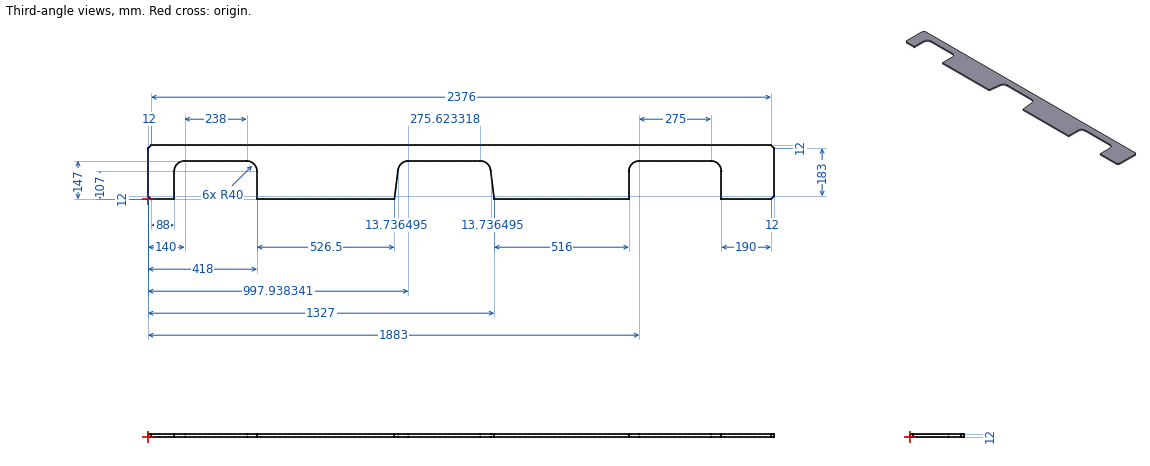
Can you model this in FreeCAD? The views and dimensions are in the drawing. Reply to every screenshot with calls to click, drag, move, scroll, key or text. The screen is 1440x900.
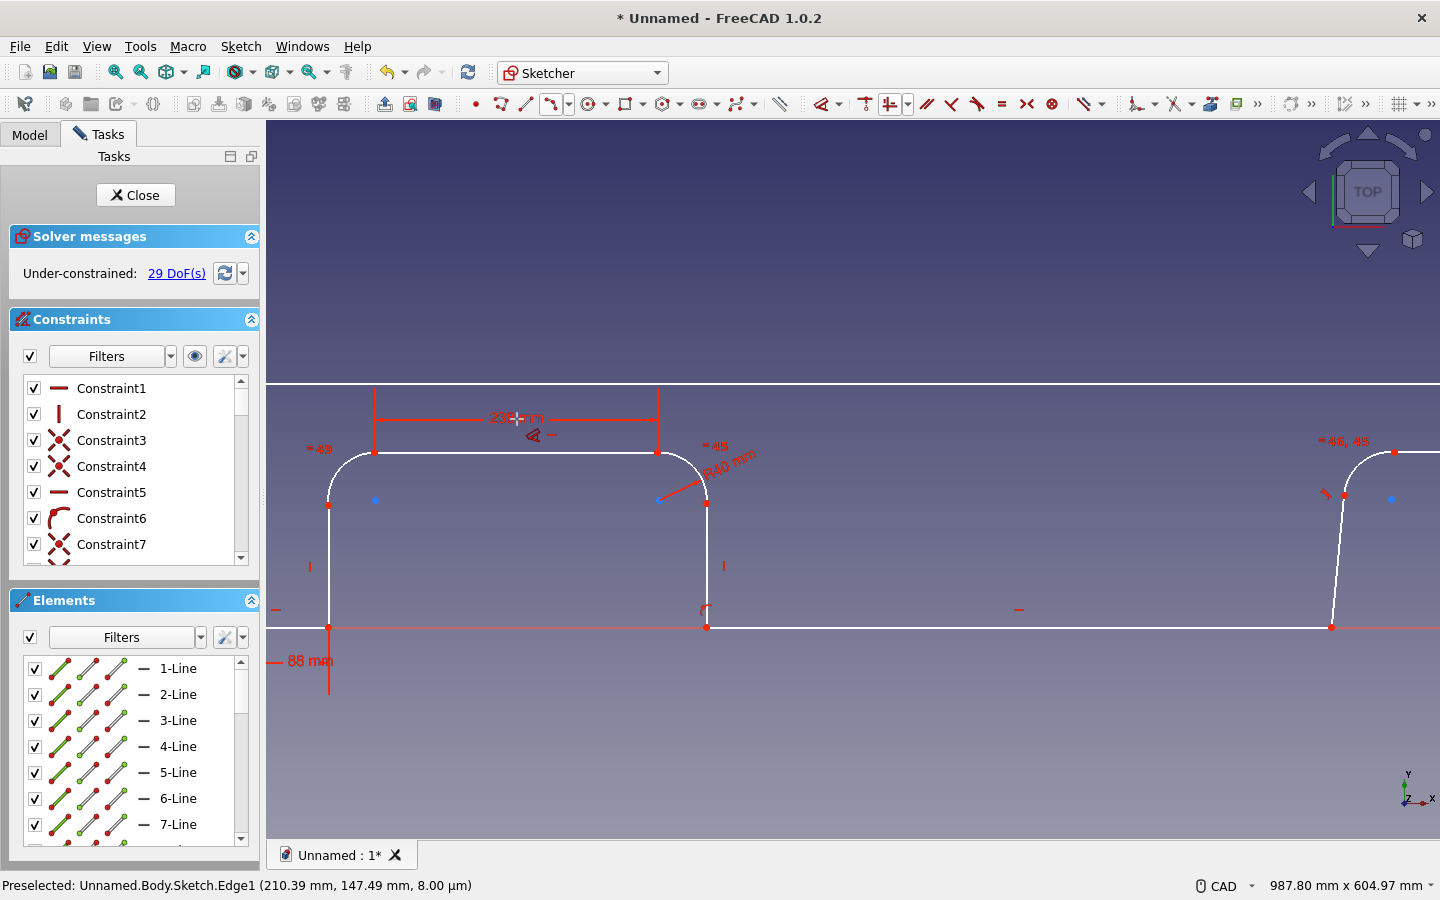
click(707, 540)
click(673, 565)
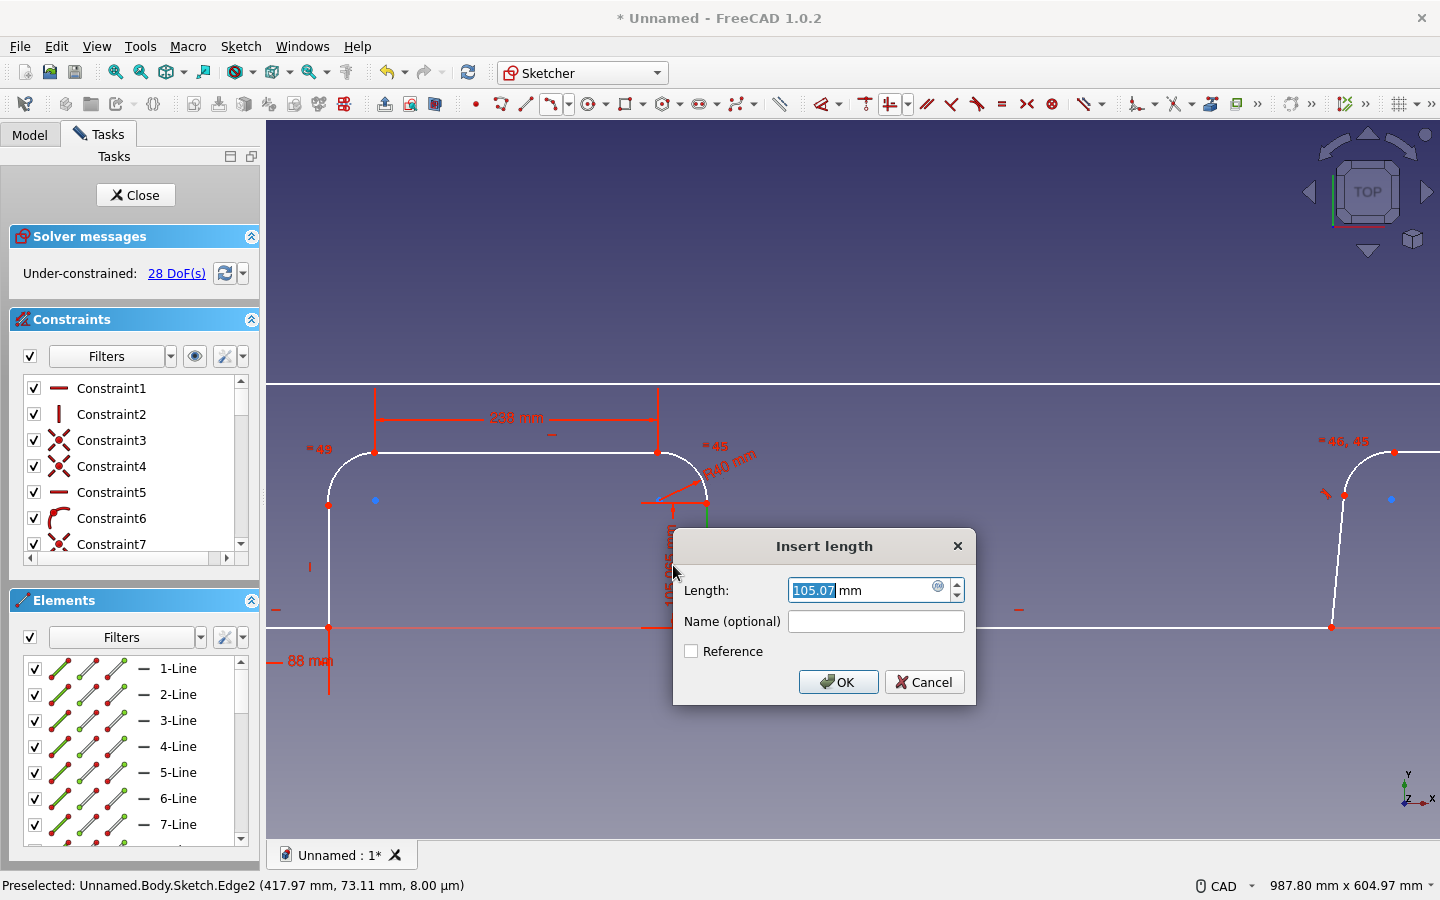
text(107)
key(Return)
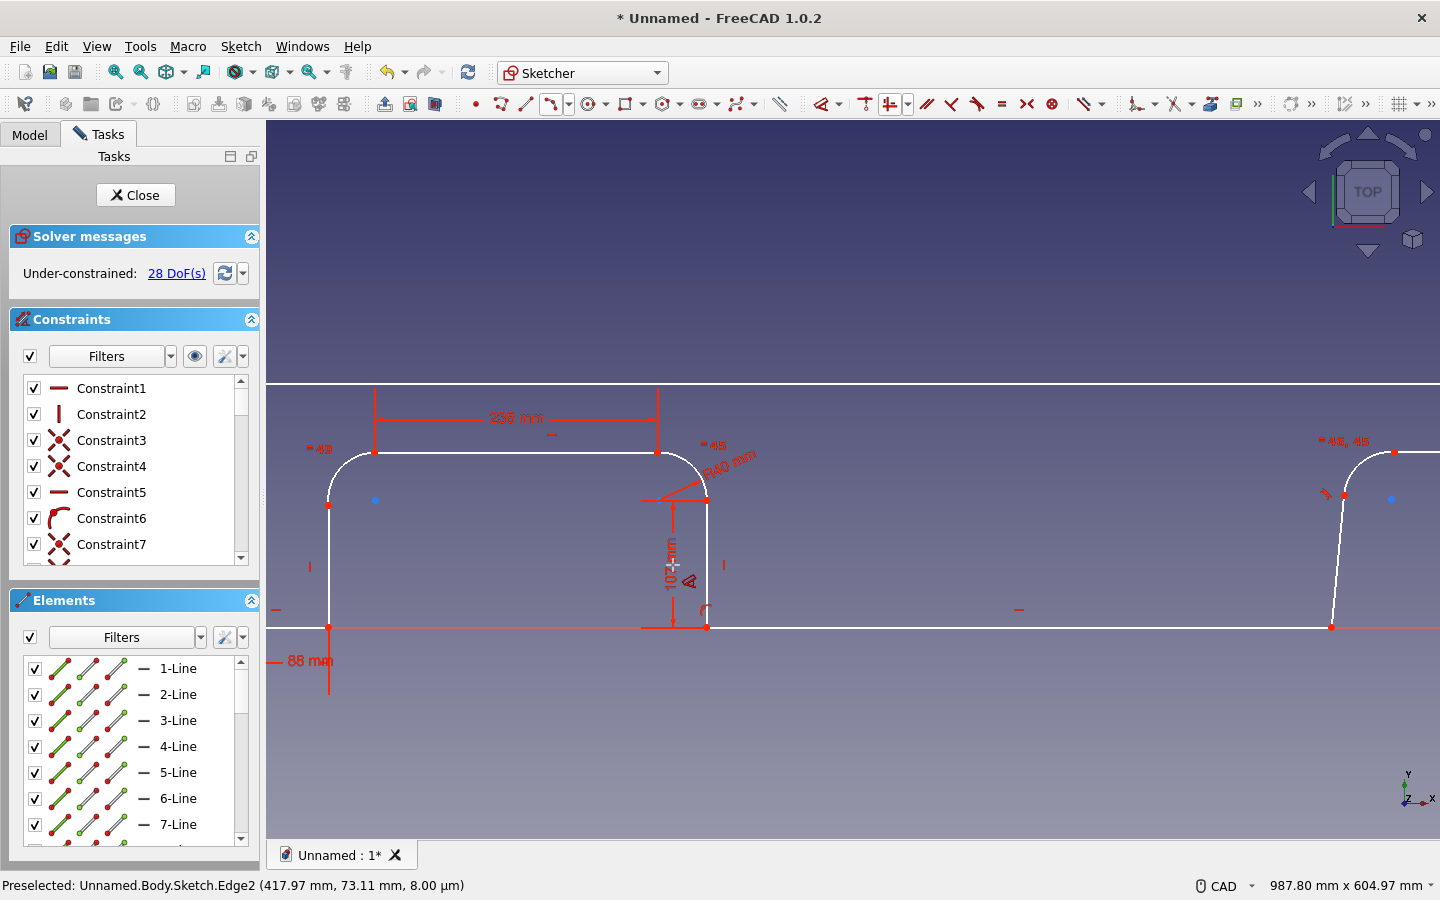
scroll(506, 471, down, 7)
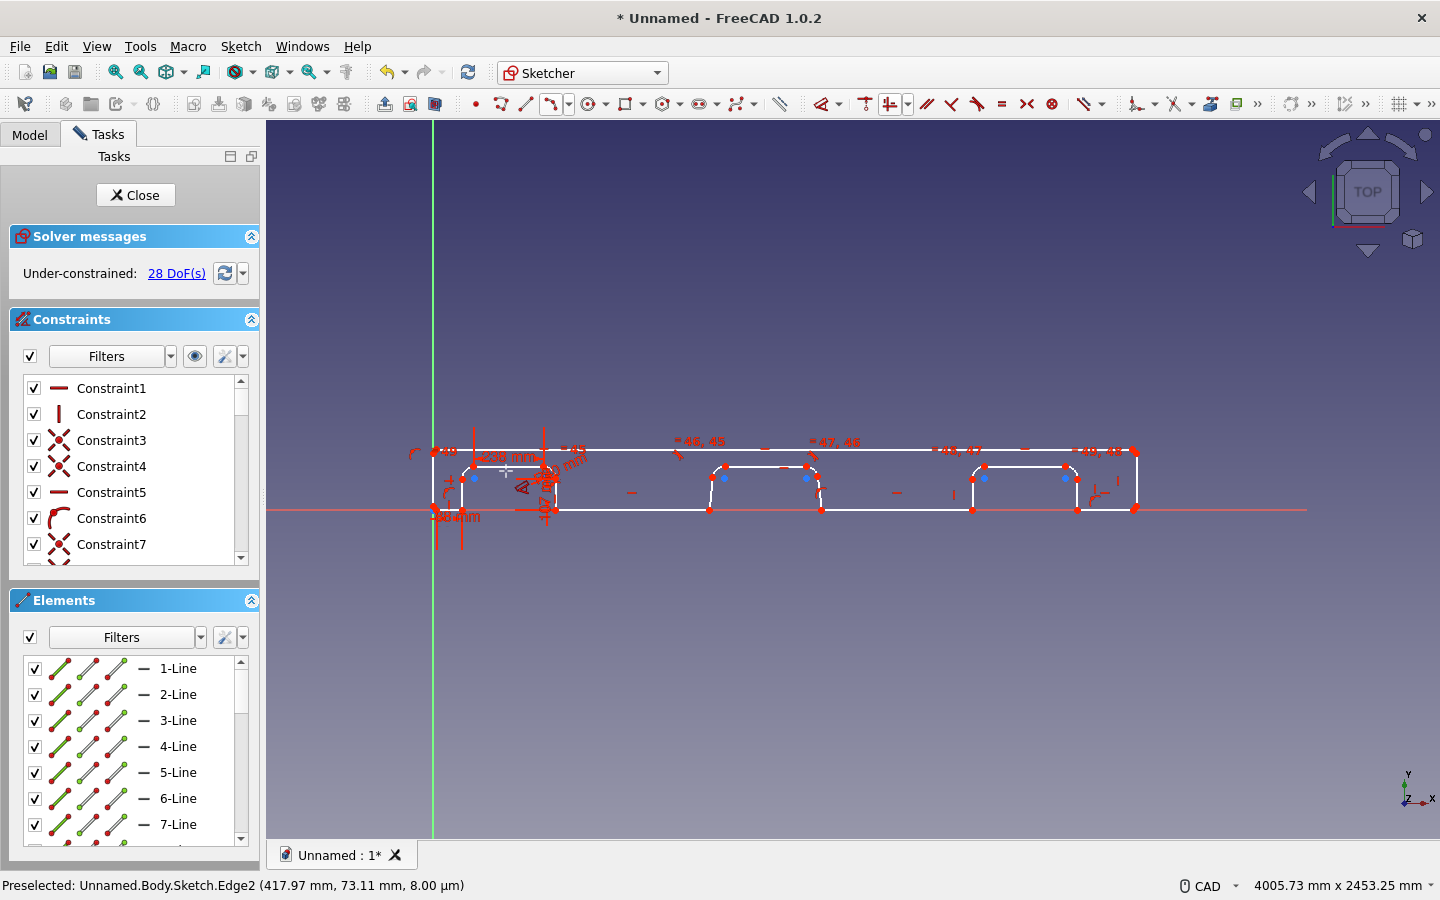
click(867, 510)
click(897, 544)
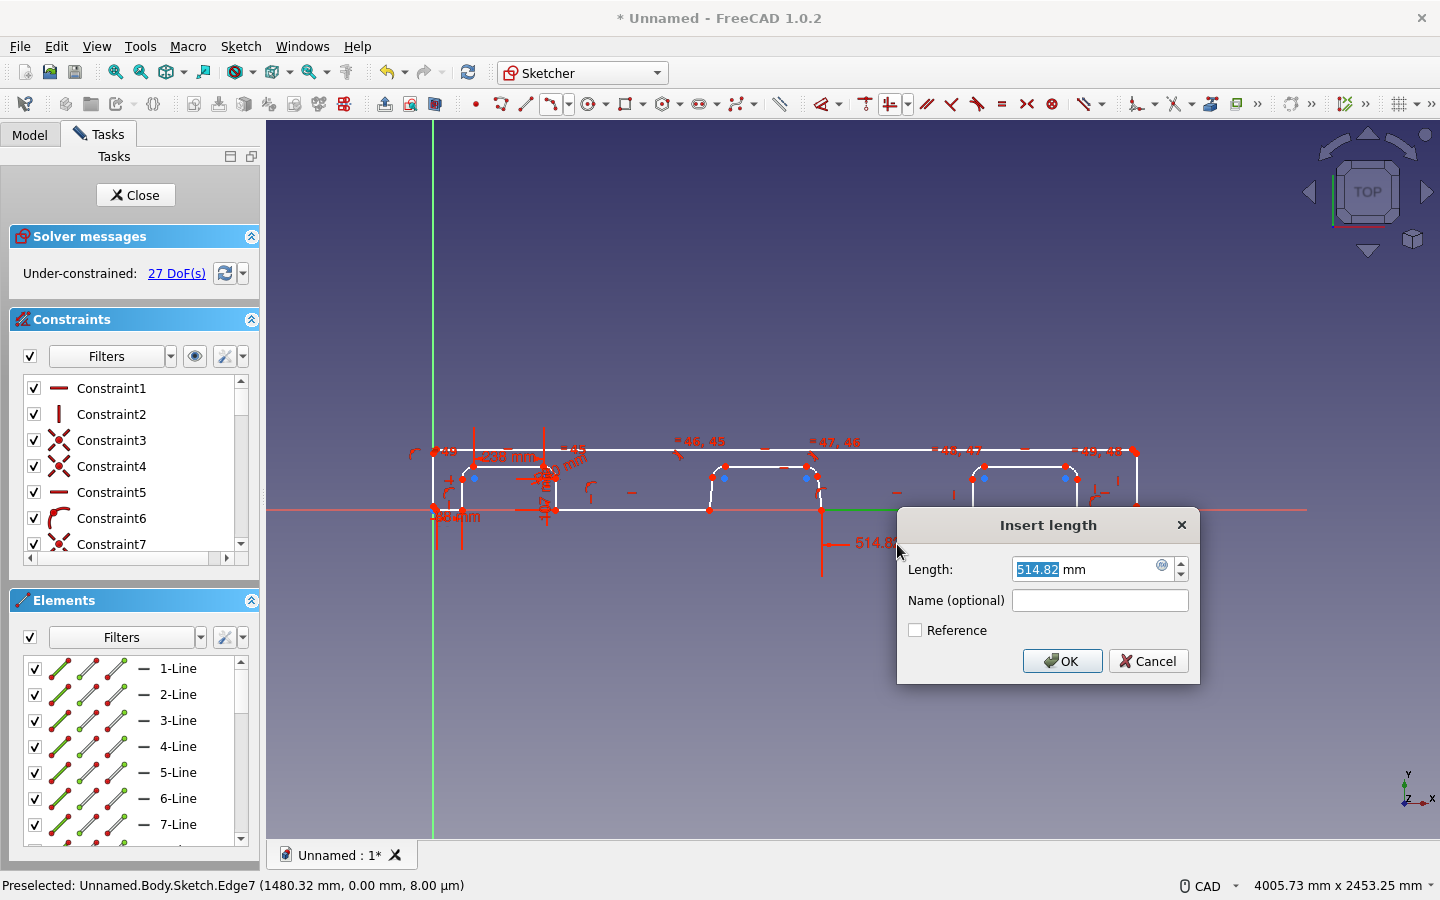
text(516)
key(Return)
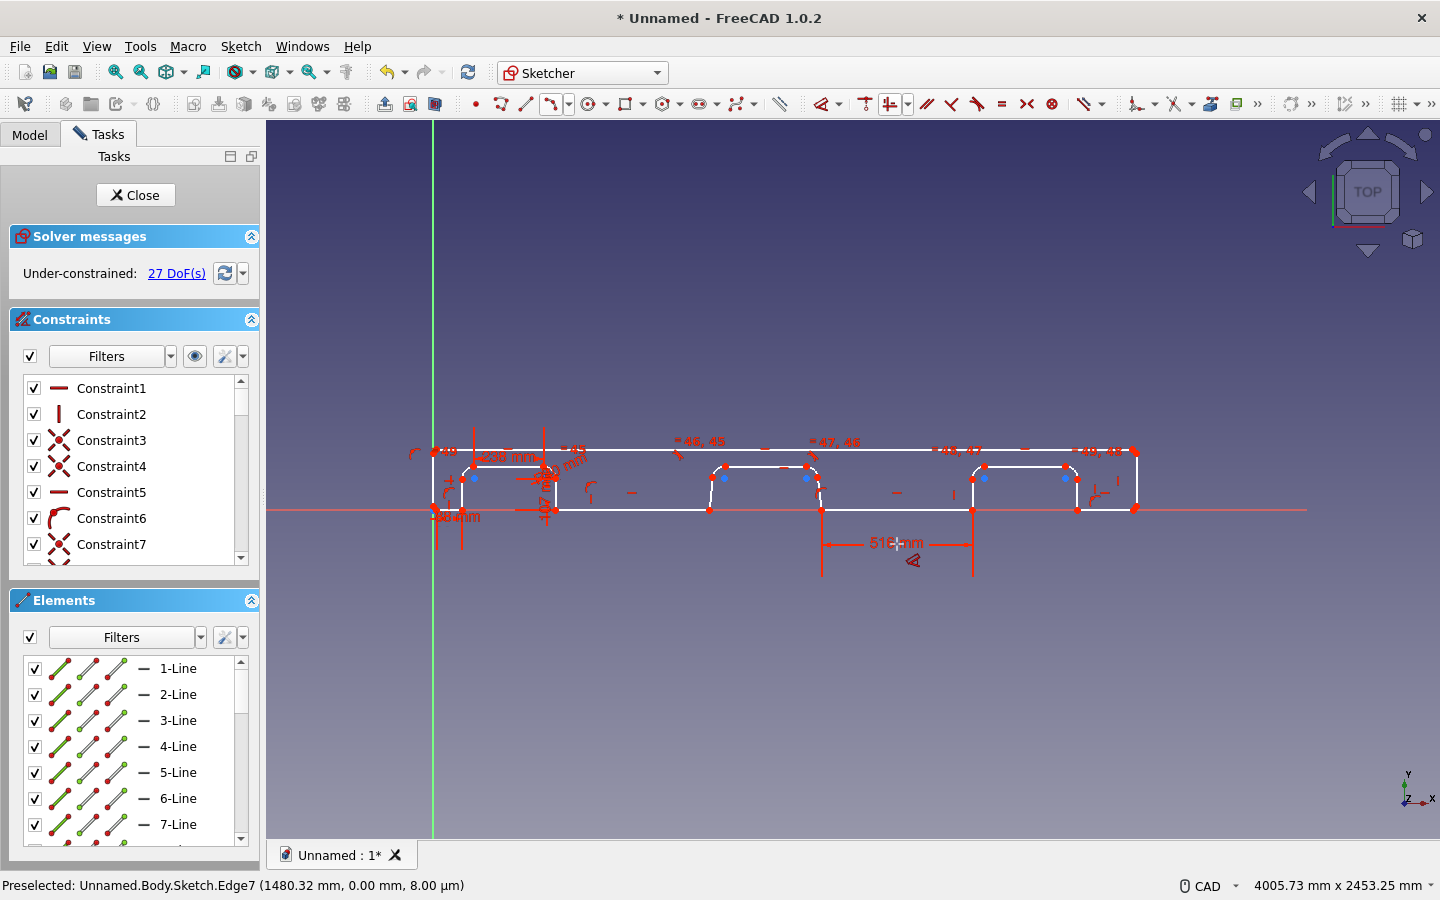
scroll(973, 501, up, 3)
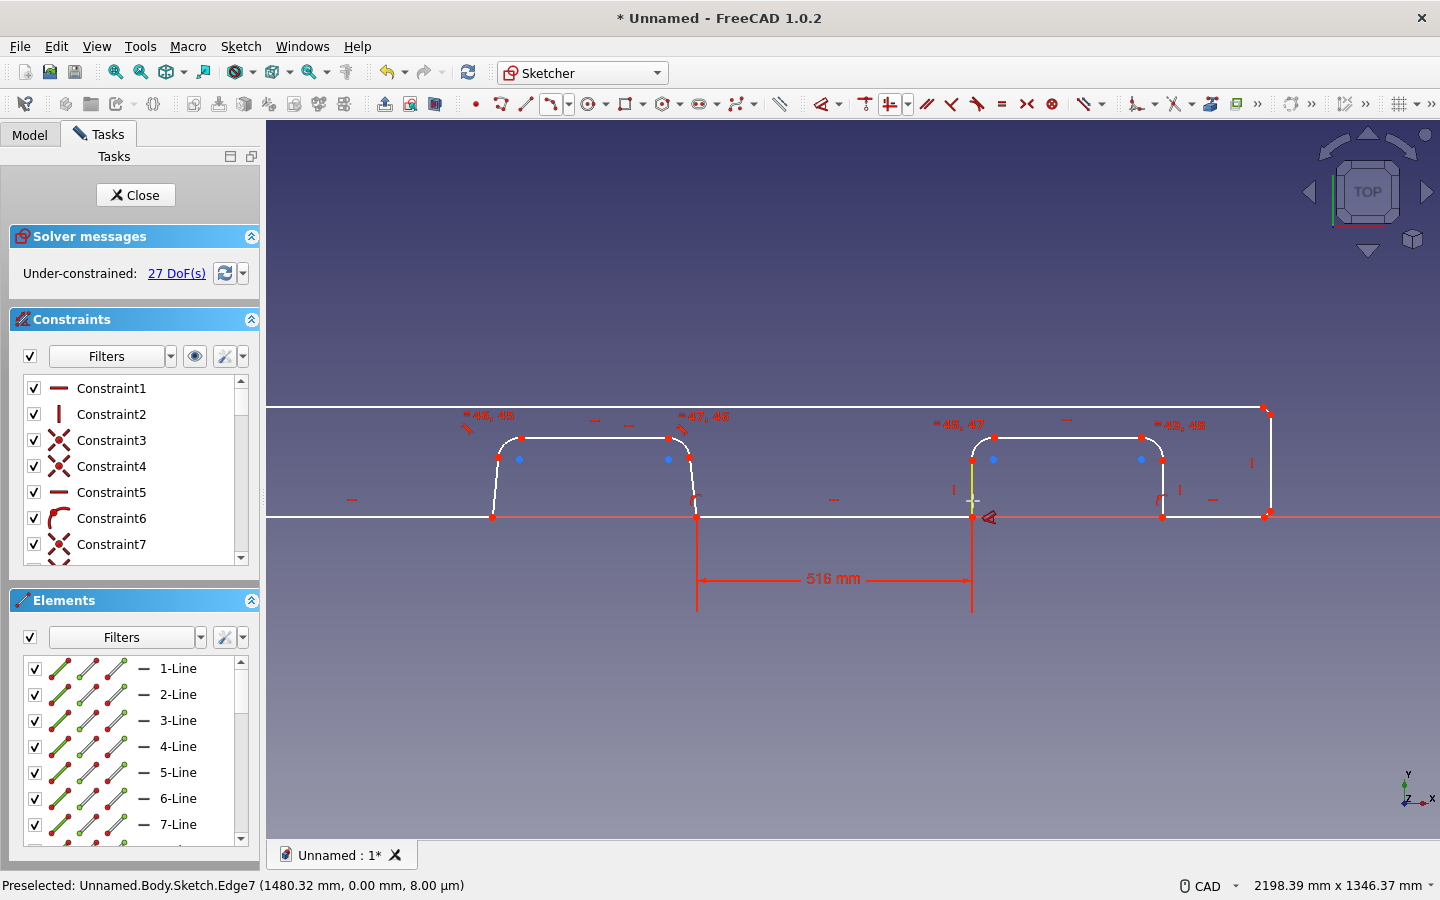
click(972, 500)
click(1006, 489)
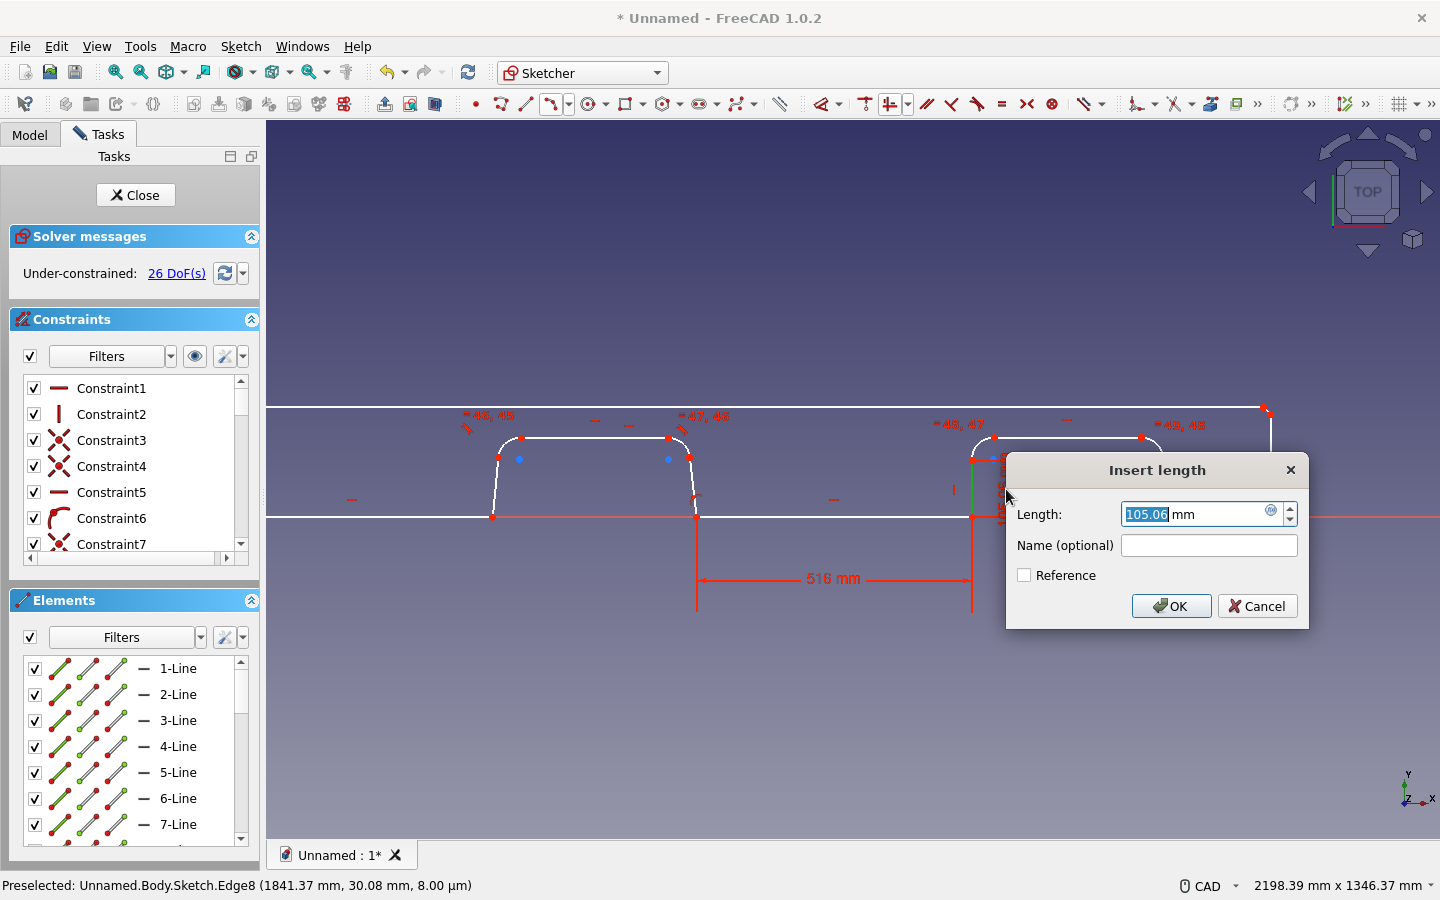
text(107)
key(Return)